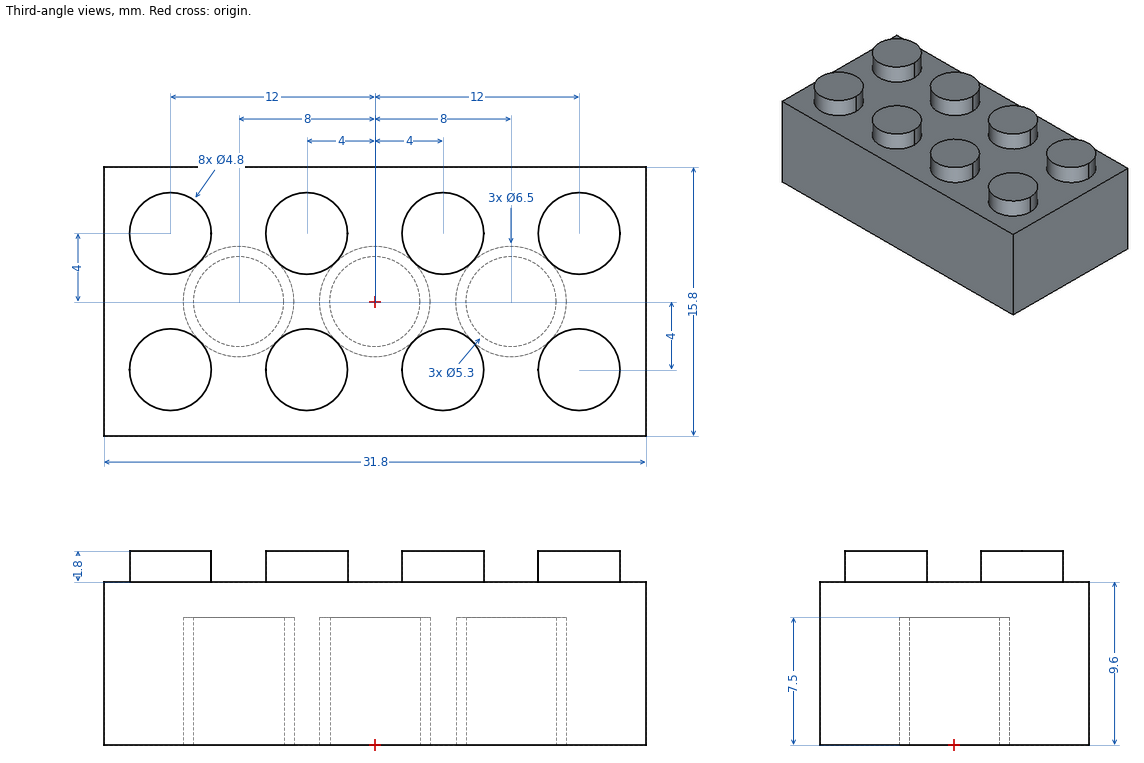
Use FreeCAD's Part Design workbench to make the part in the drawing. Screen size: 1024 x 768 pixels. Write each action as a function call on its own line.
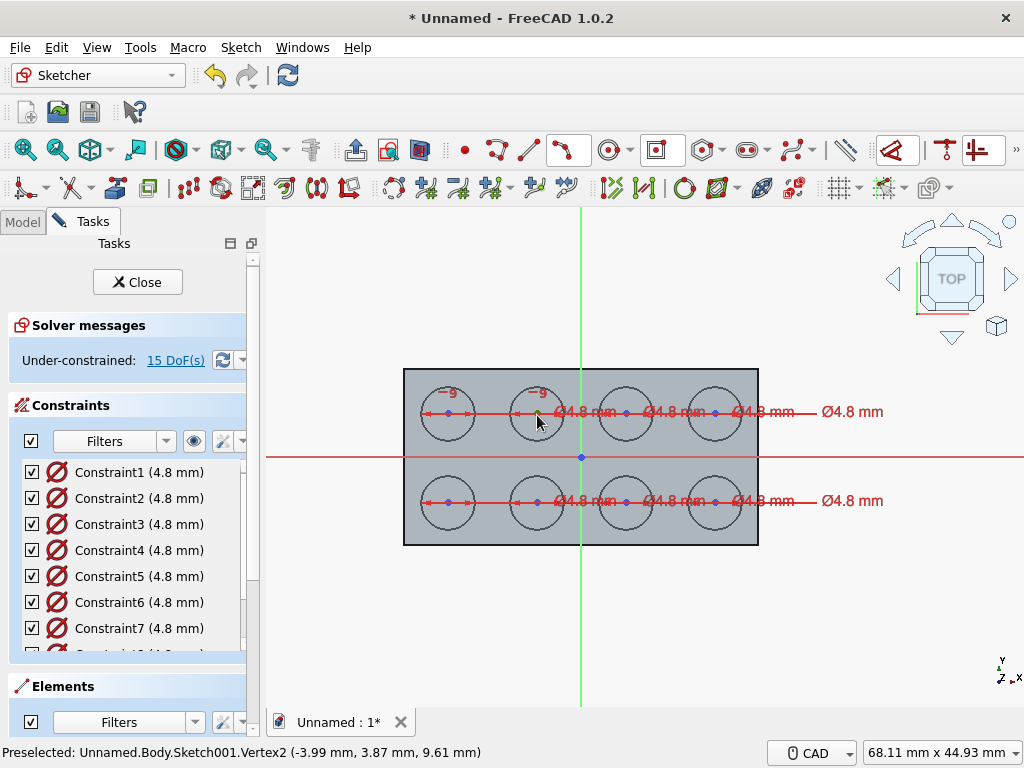
click(626, 414)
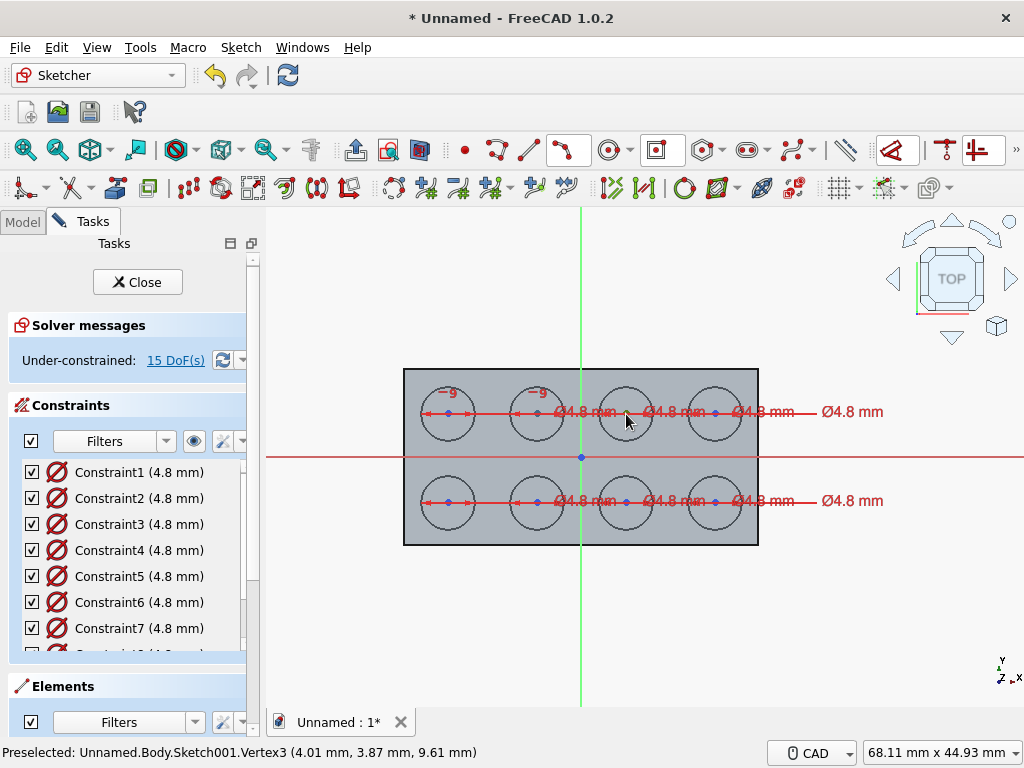
key(h)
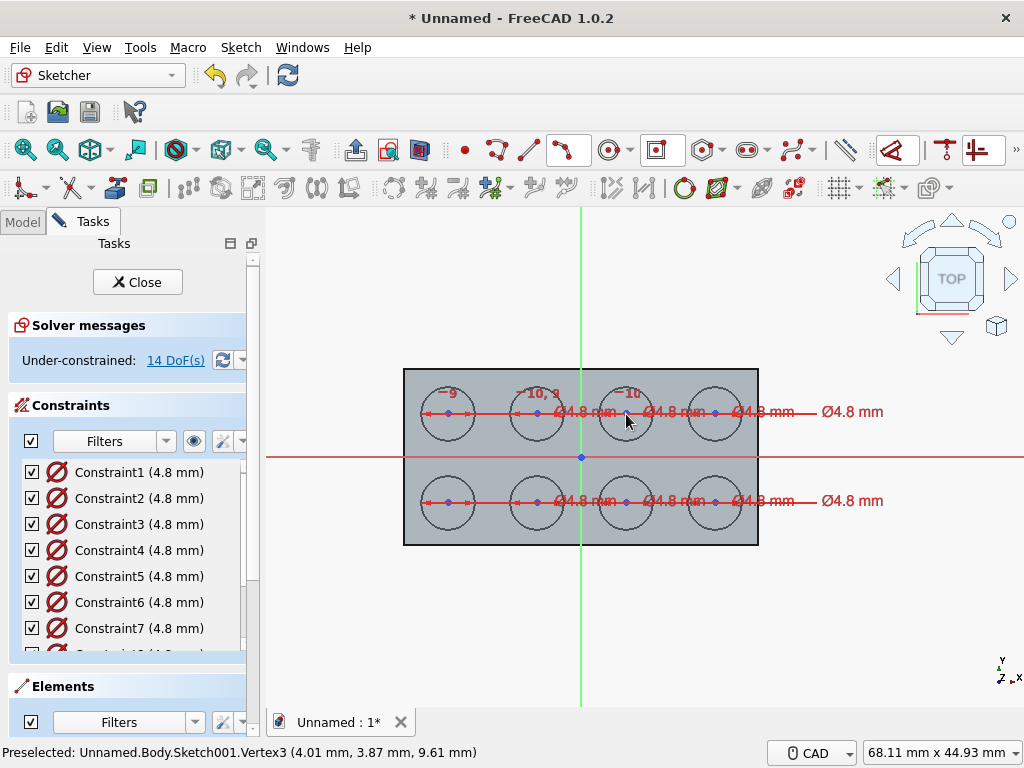
click(626, 414)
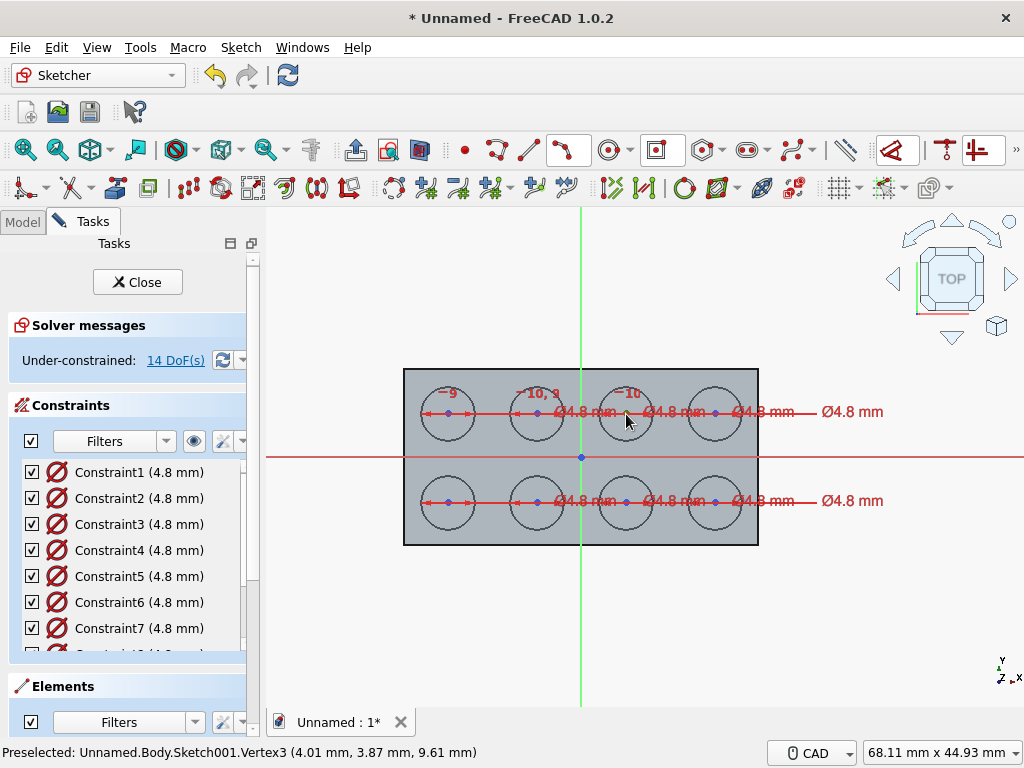
click(715, 414)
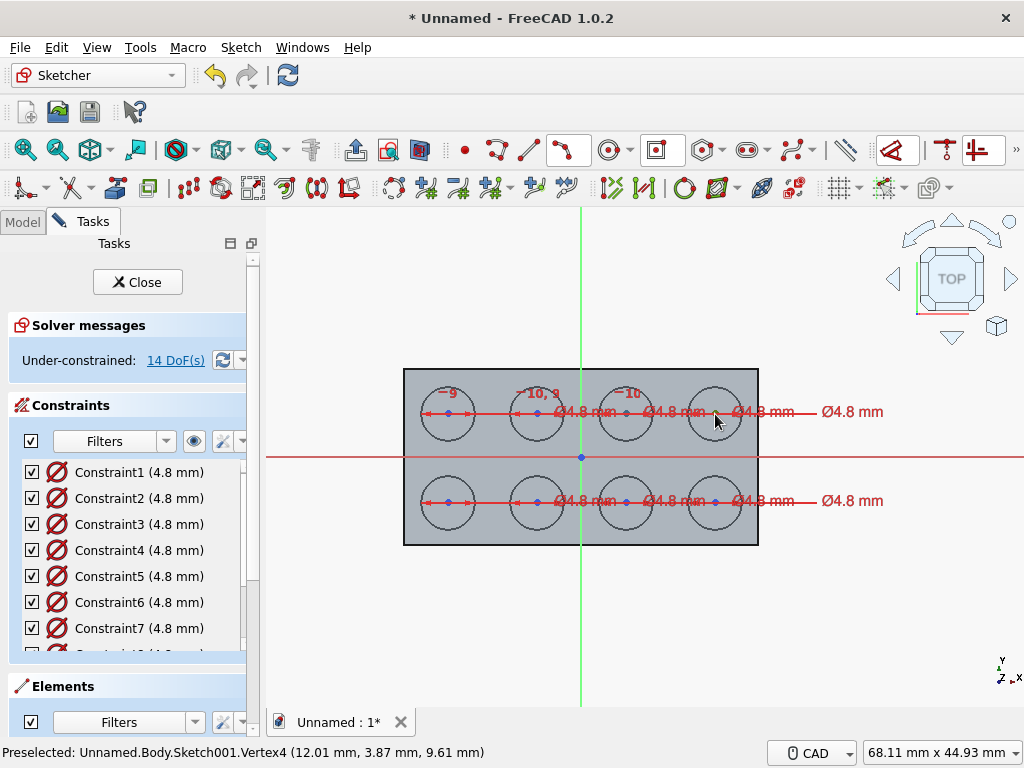
click(1000, 150)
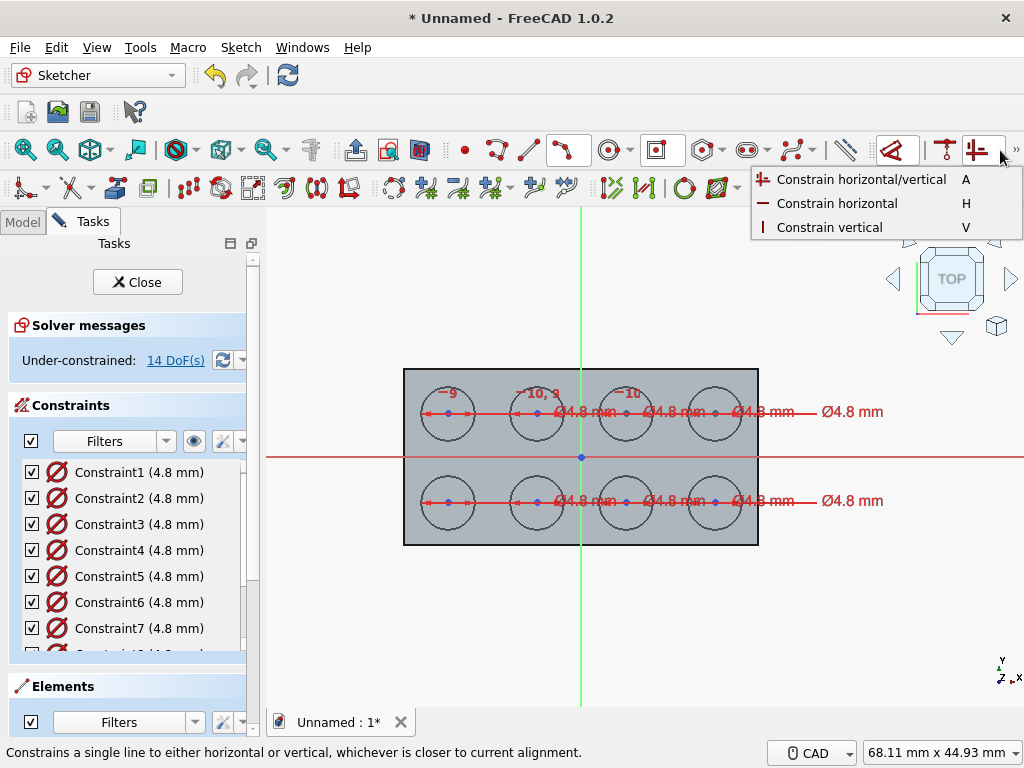
click(887, 203)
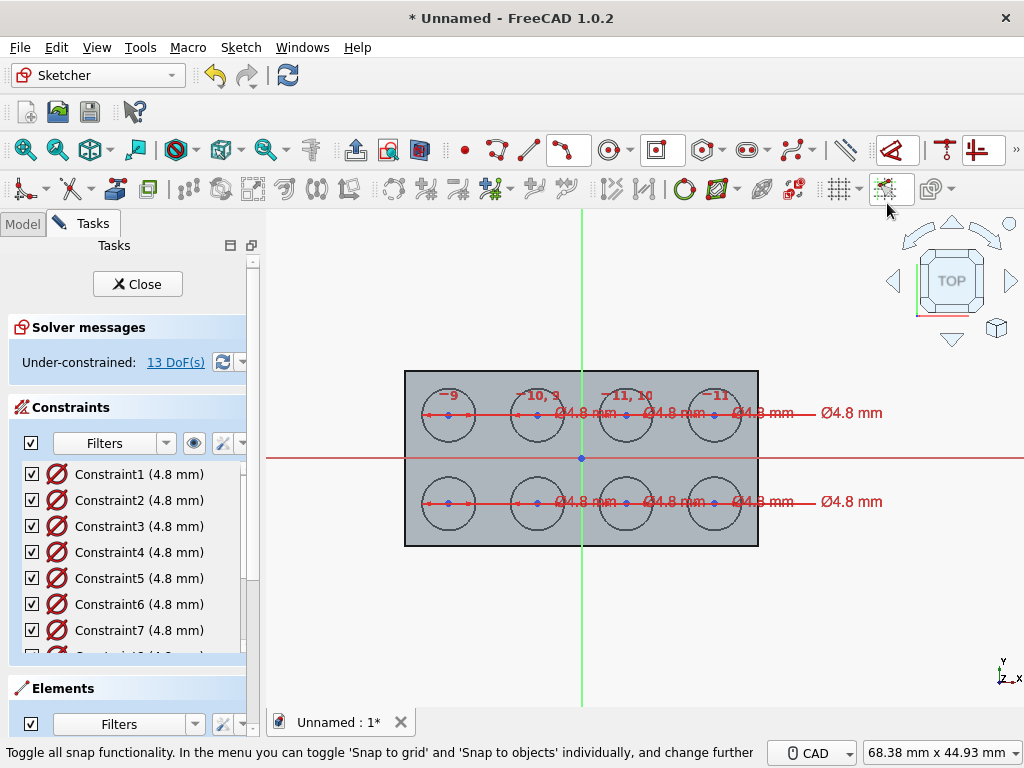
click(715, 415)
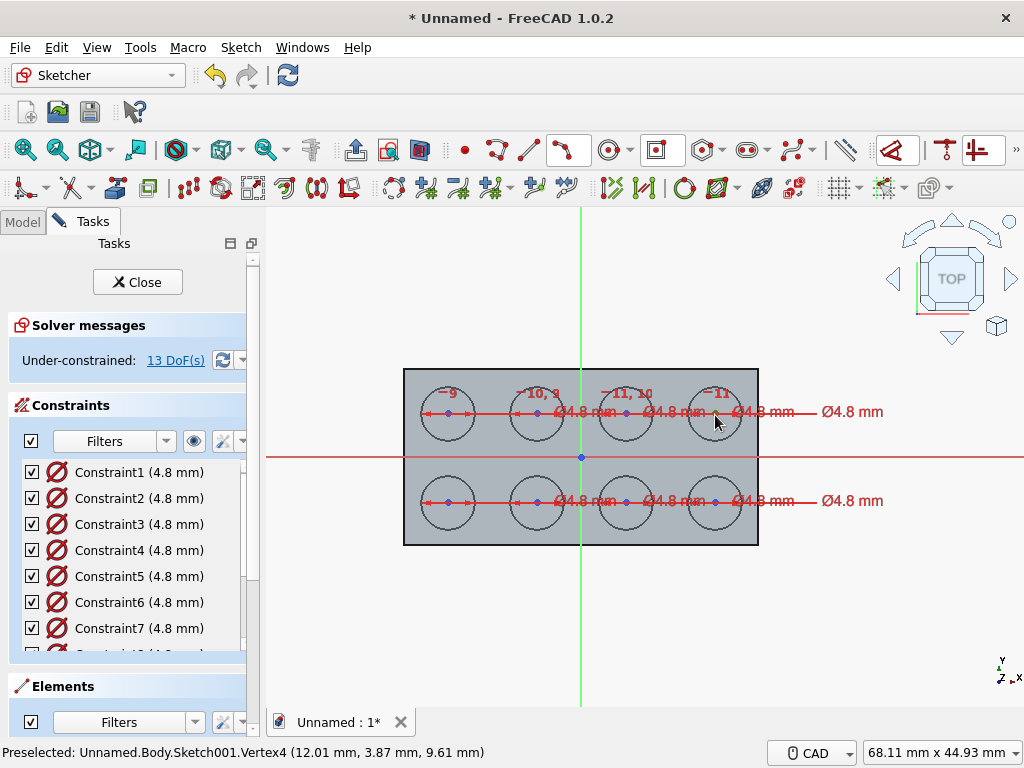
click(715, 503)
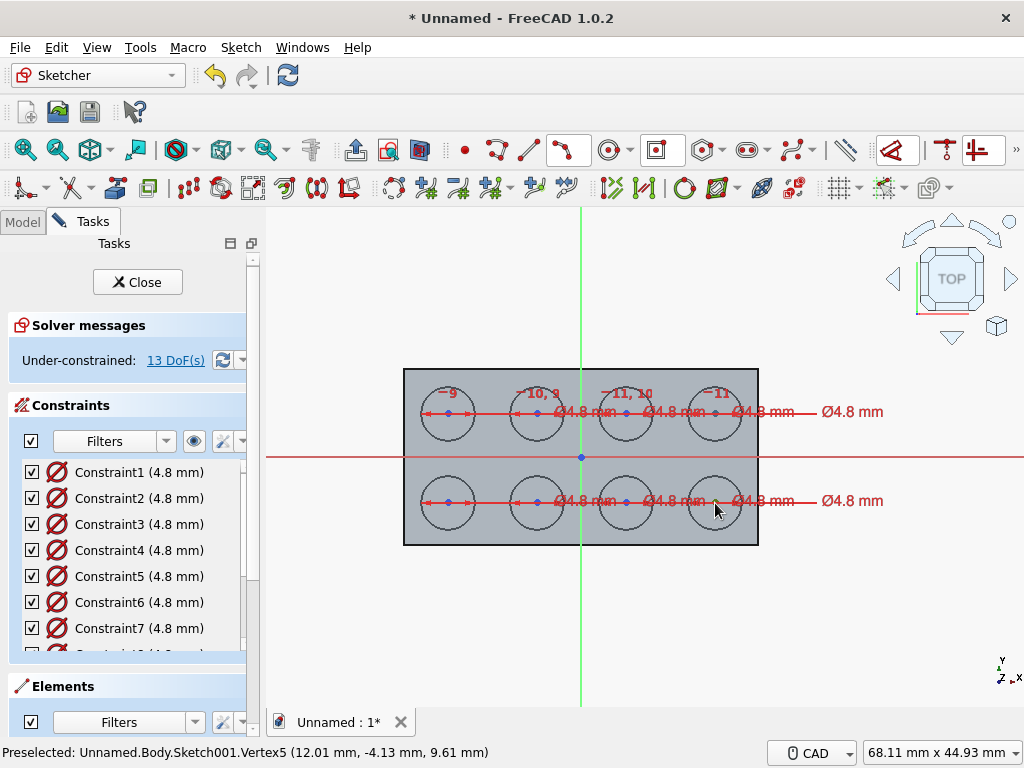
click(1000, 150)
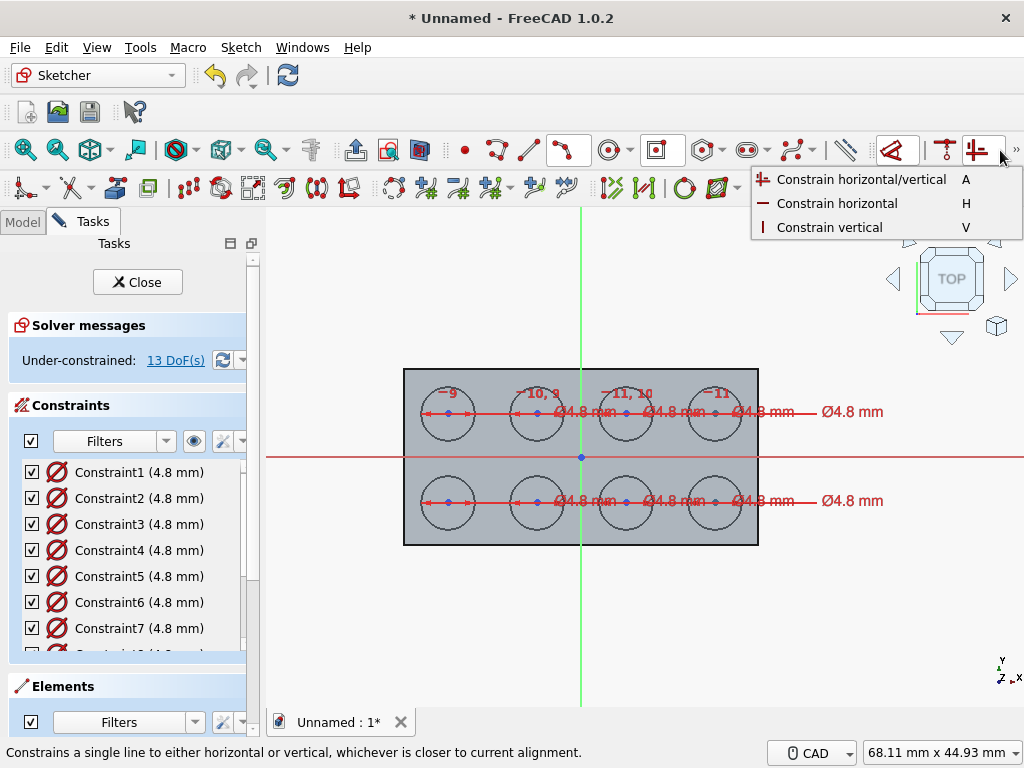
click(887, 227)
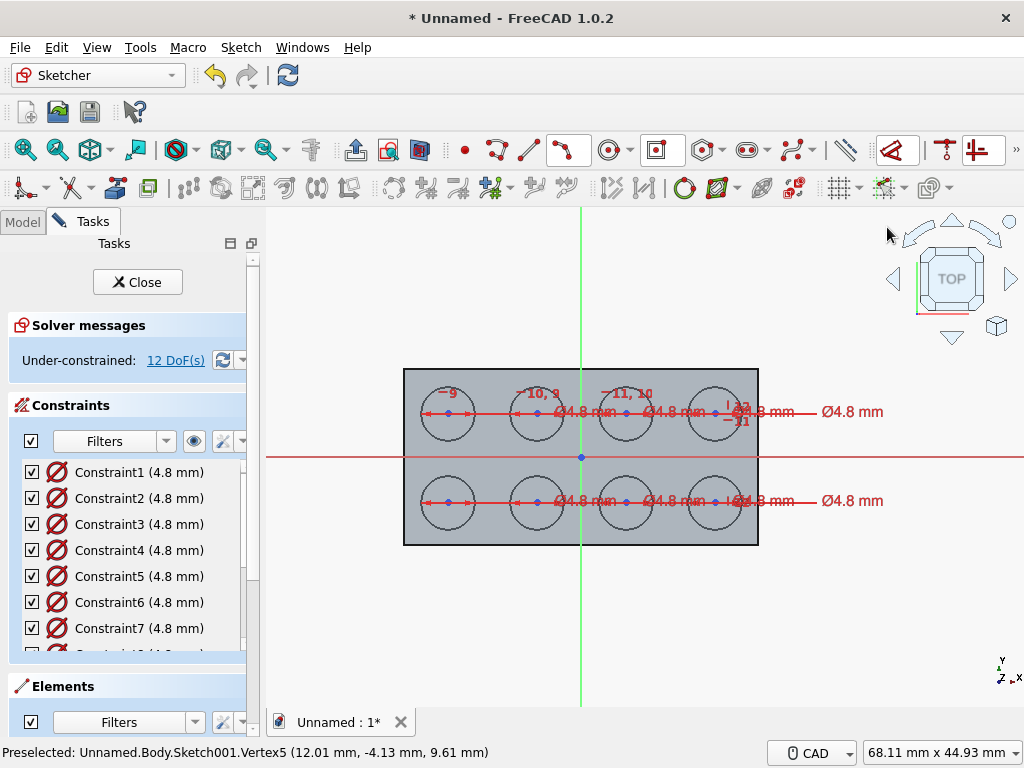
click(626, 414)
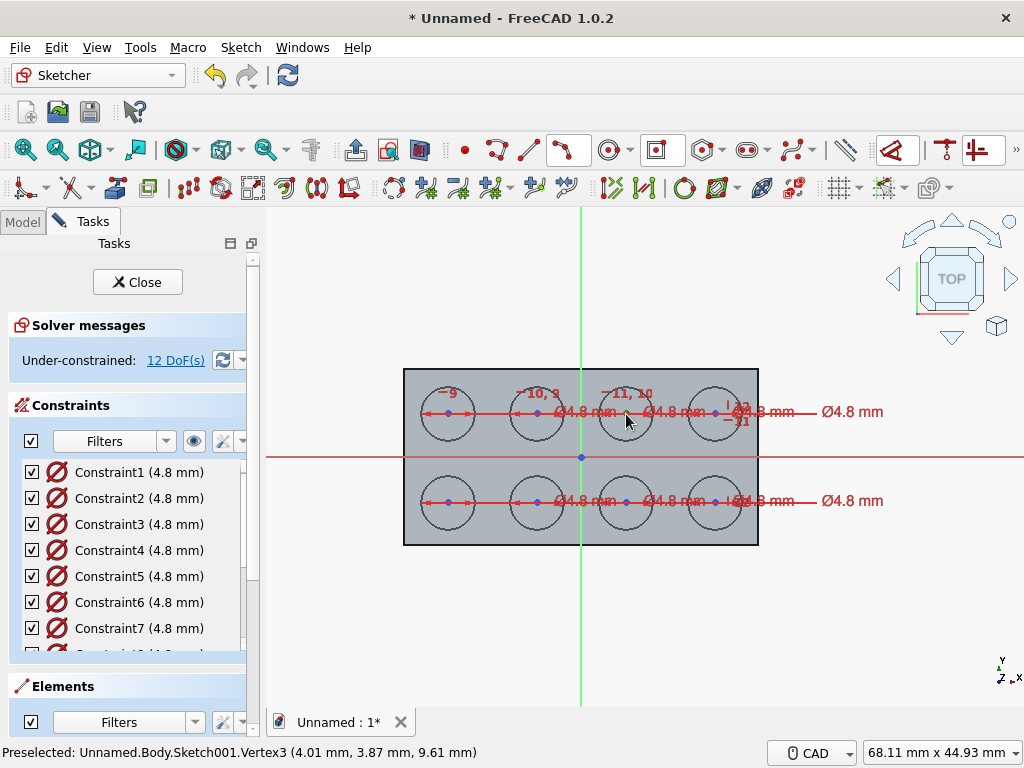
click(626, 503)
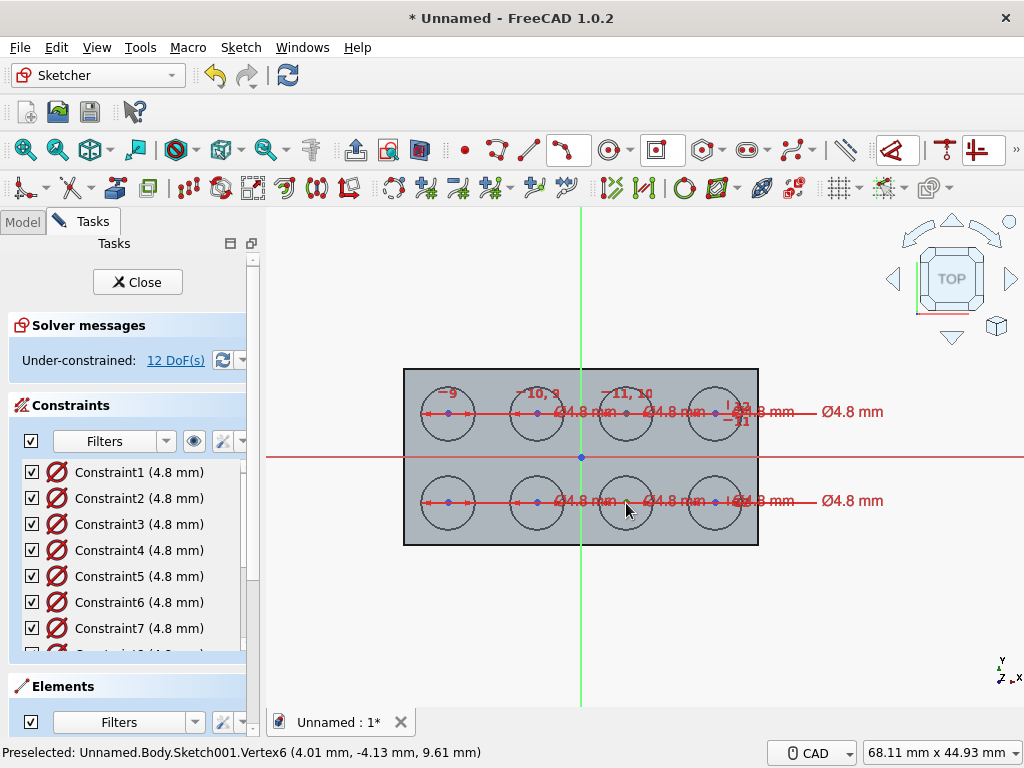
key(v)